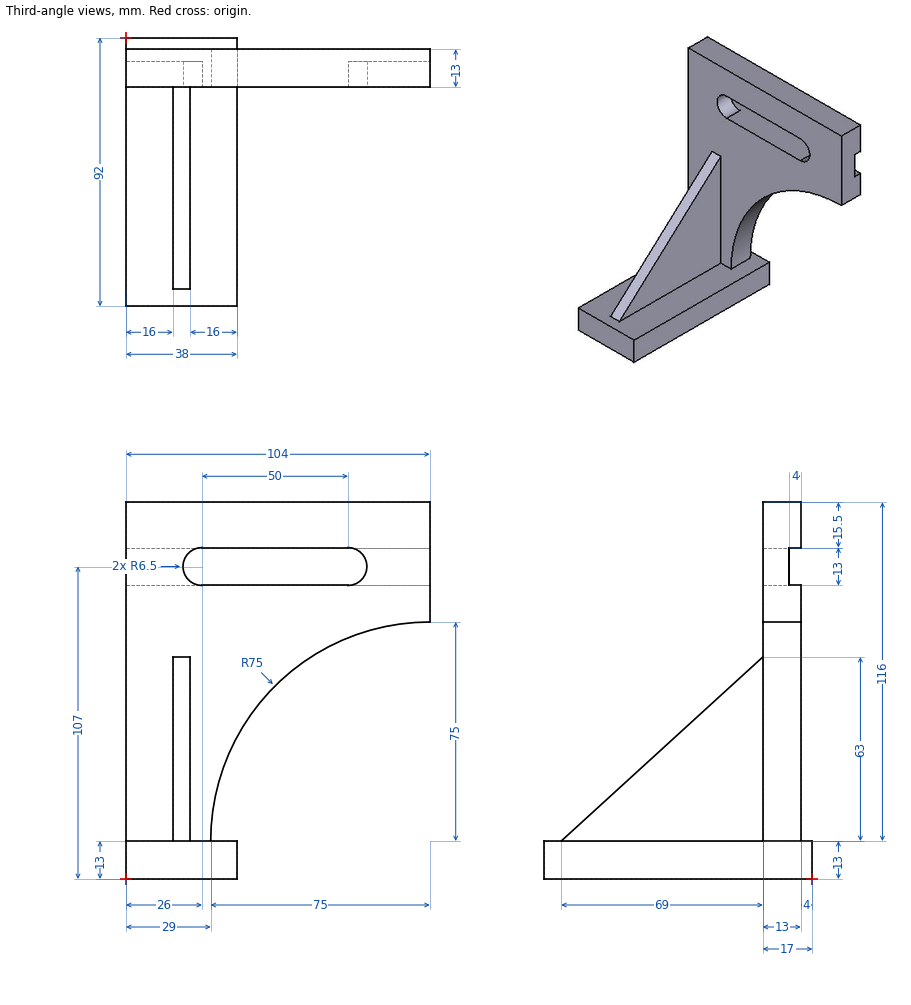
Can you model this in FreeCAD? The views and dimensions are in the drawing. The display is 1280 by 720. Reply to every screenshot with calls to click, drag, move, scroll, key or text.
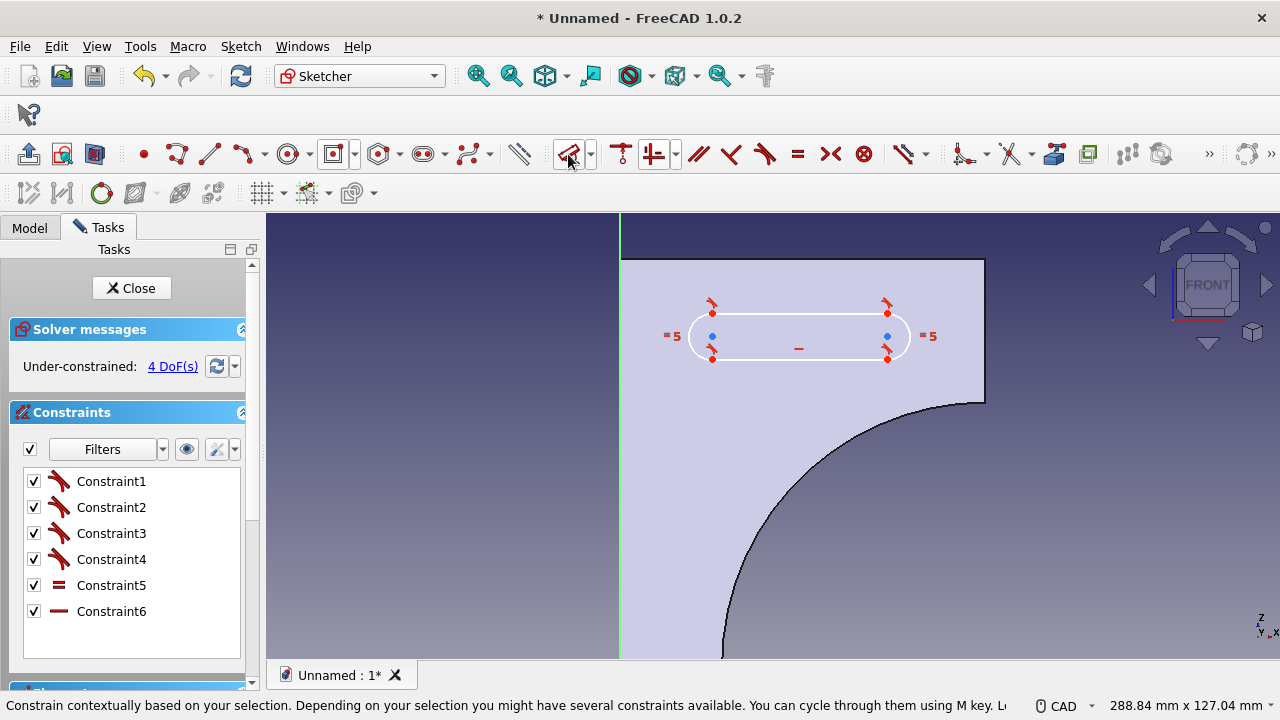
scroll(693, 323, up, 3)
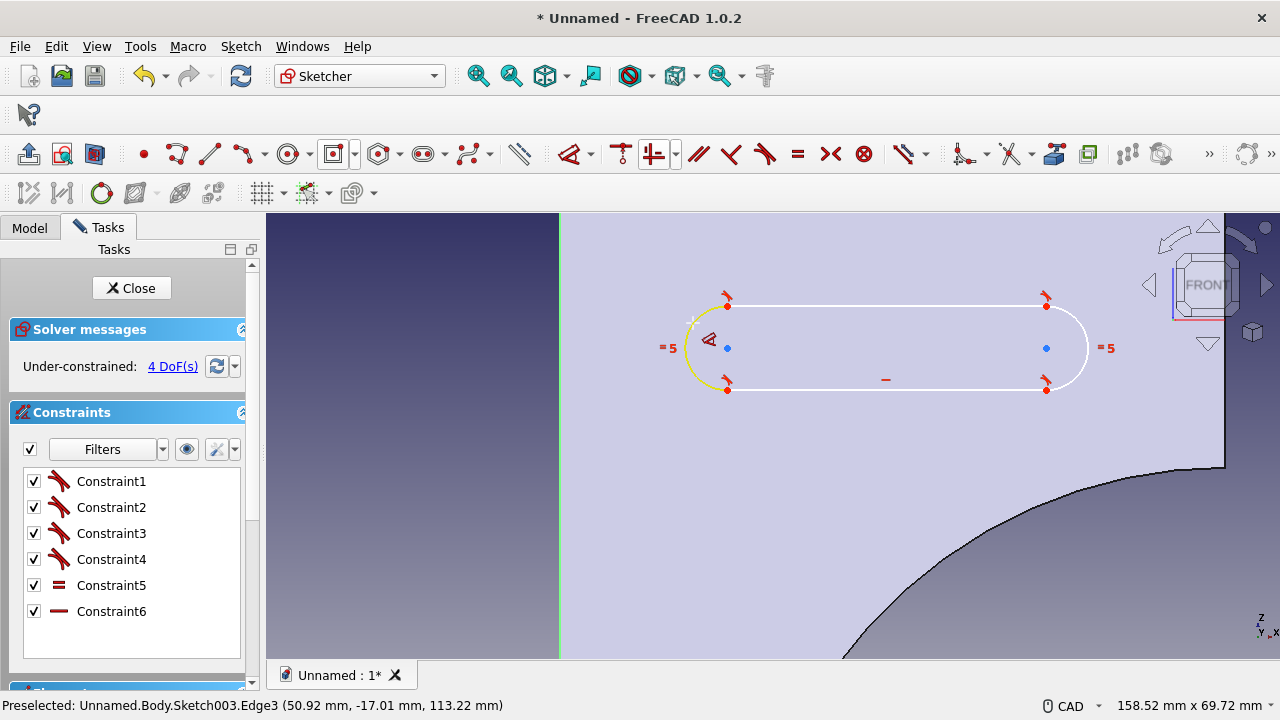
click(693, 324)
click(667, 305)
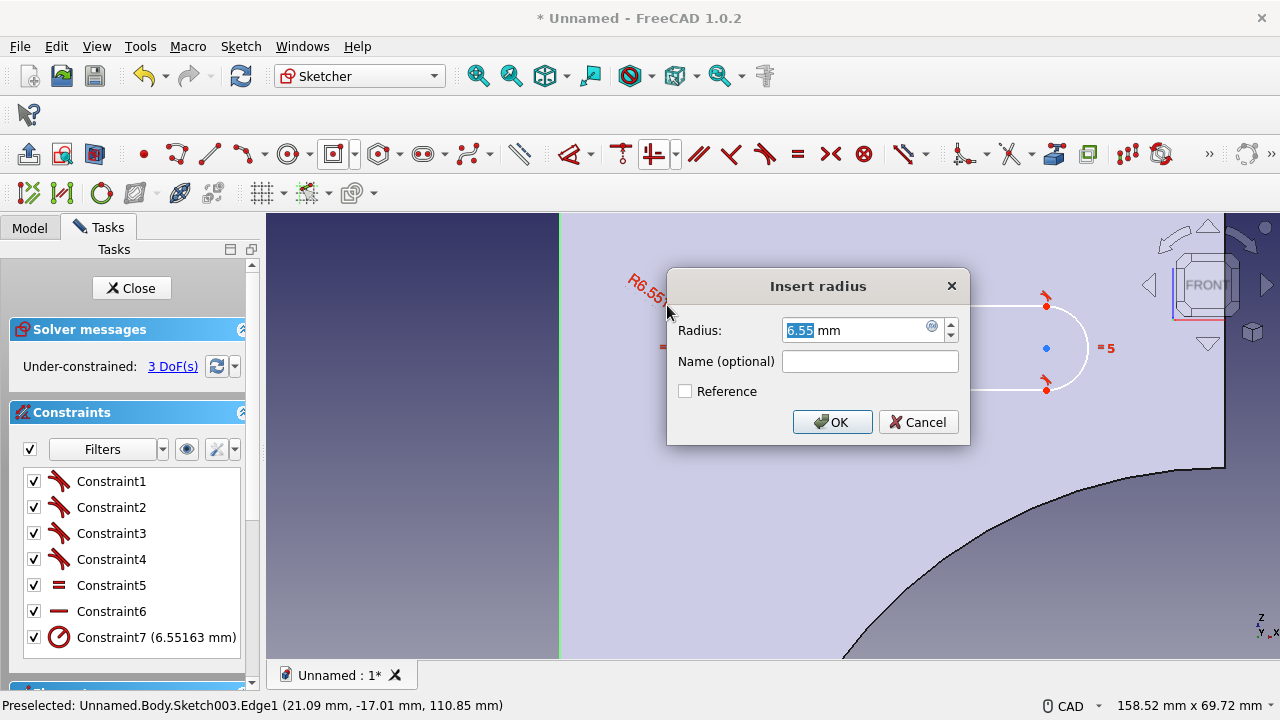
text(6.5)
key(Return)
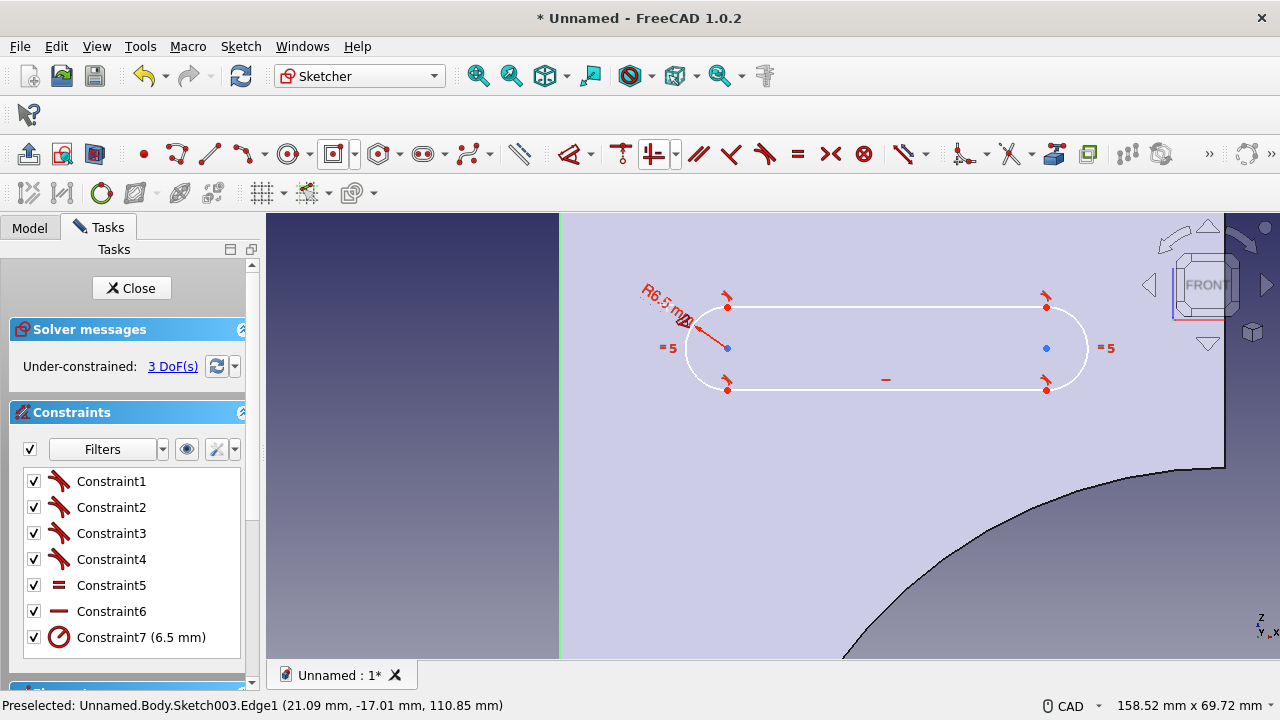
click(823, 307)
click(887, 273)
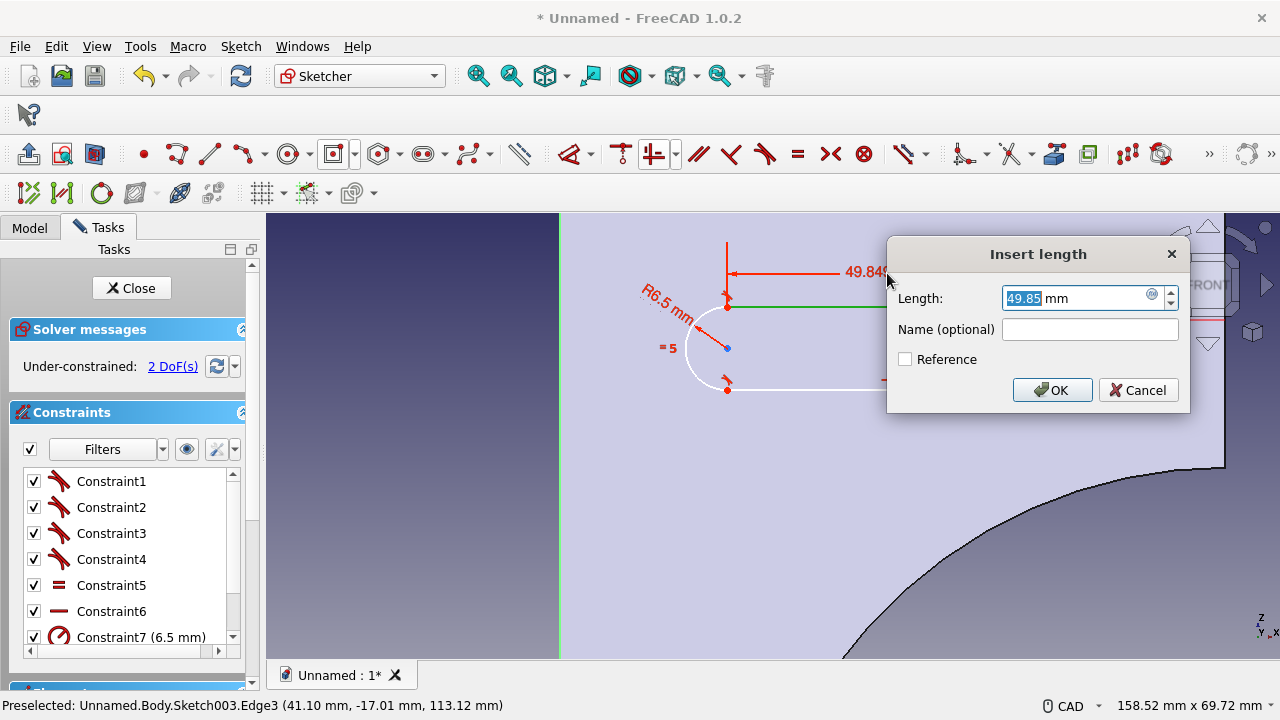
text(50)
key(Return)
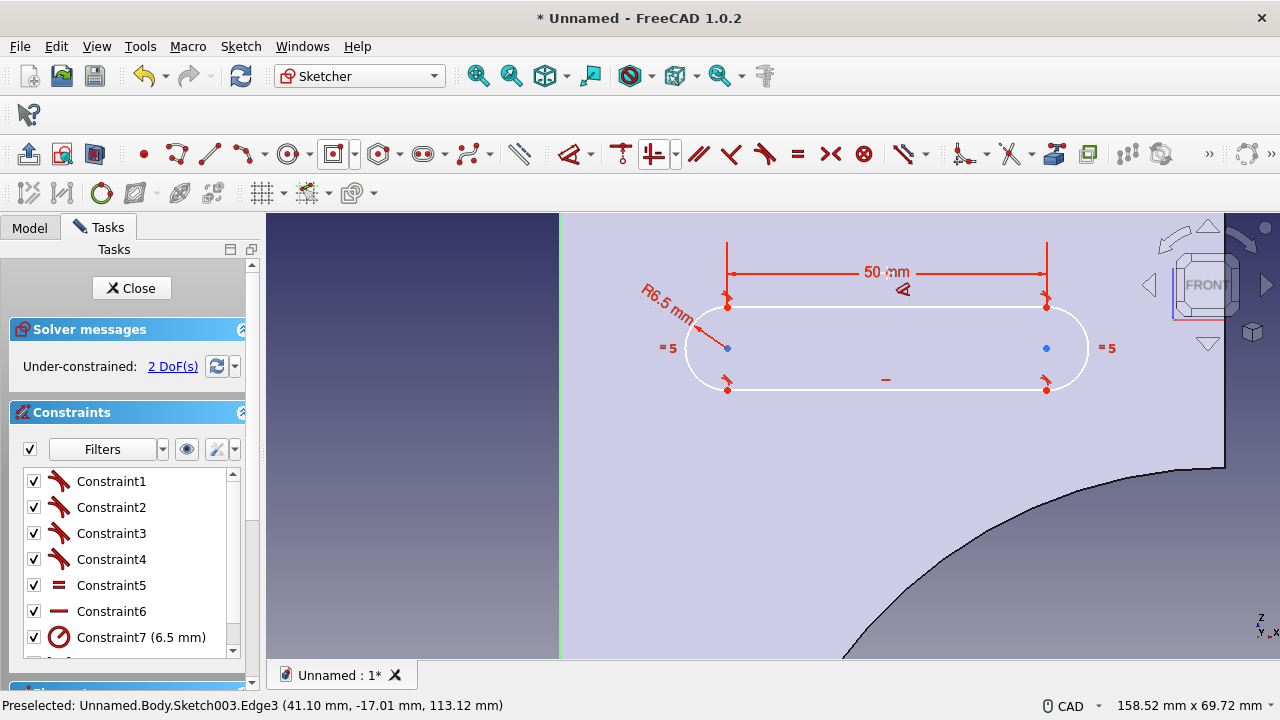
click(727, 307)
click(644, 273)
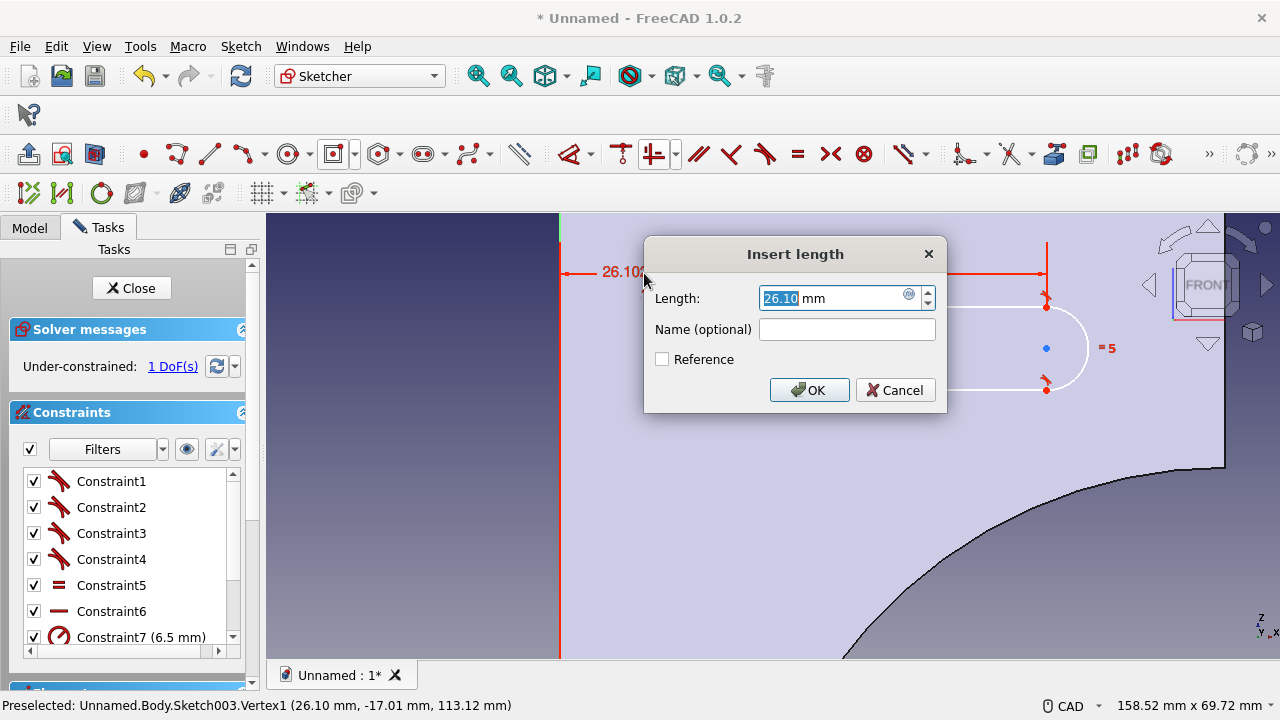
text(26)
key(Return)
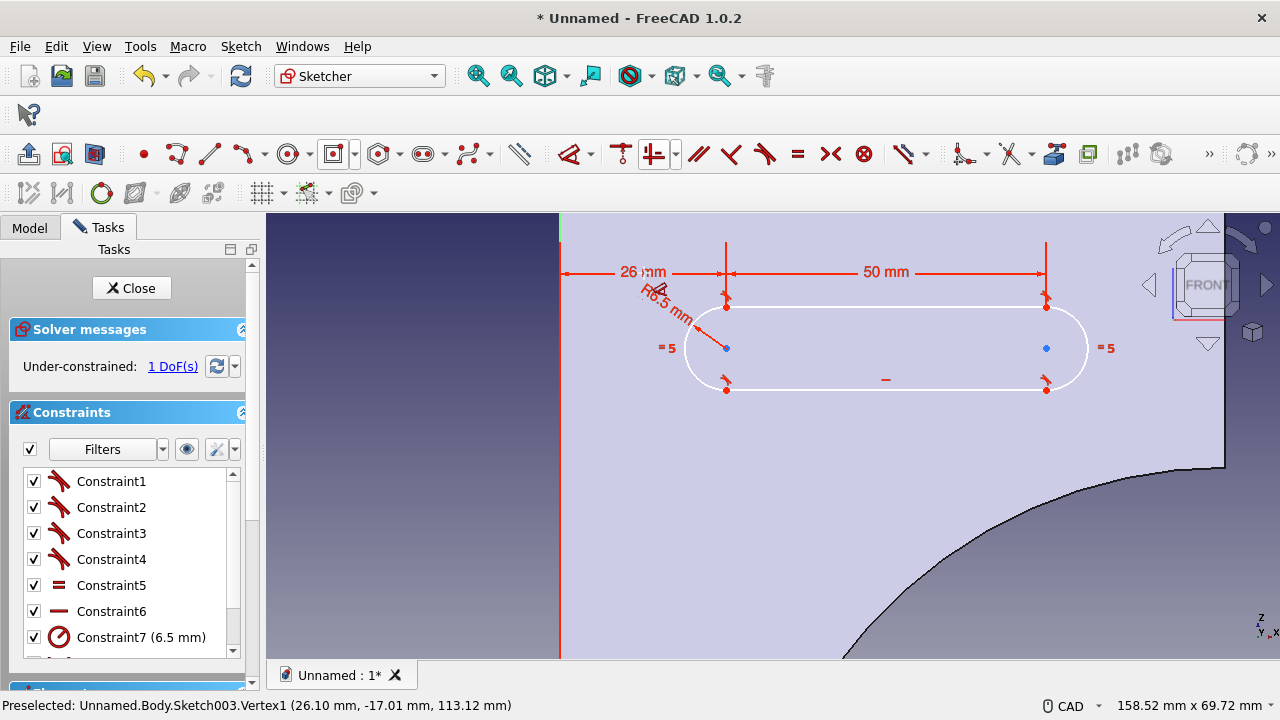
click(726, 349)
click(526, 490)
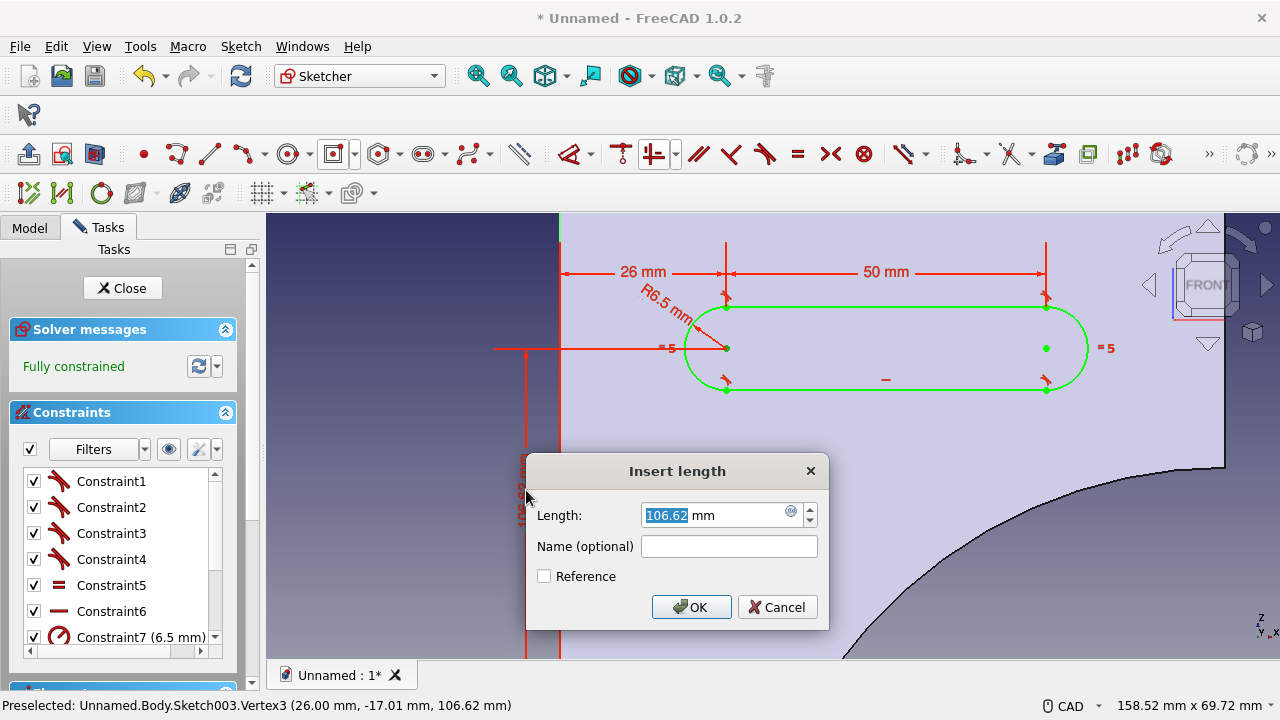
text(107)
key(Return)
key(Escape)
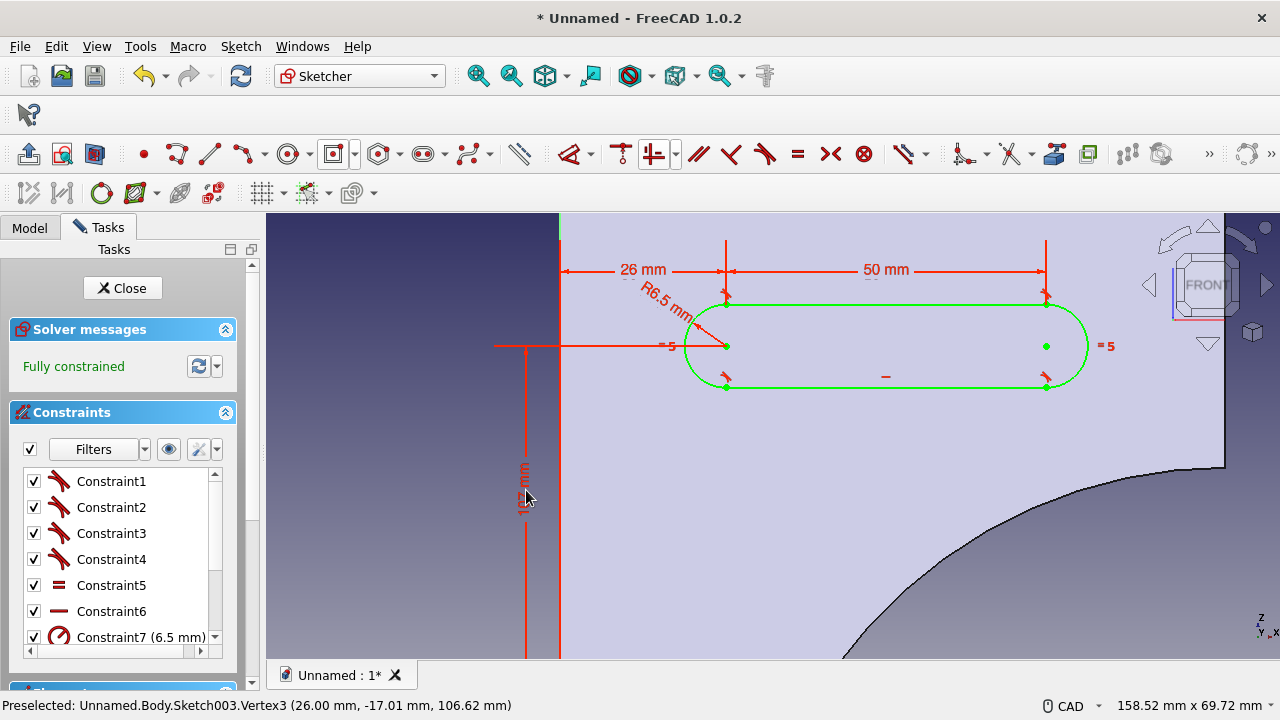
click(123, 288)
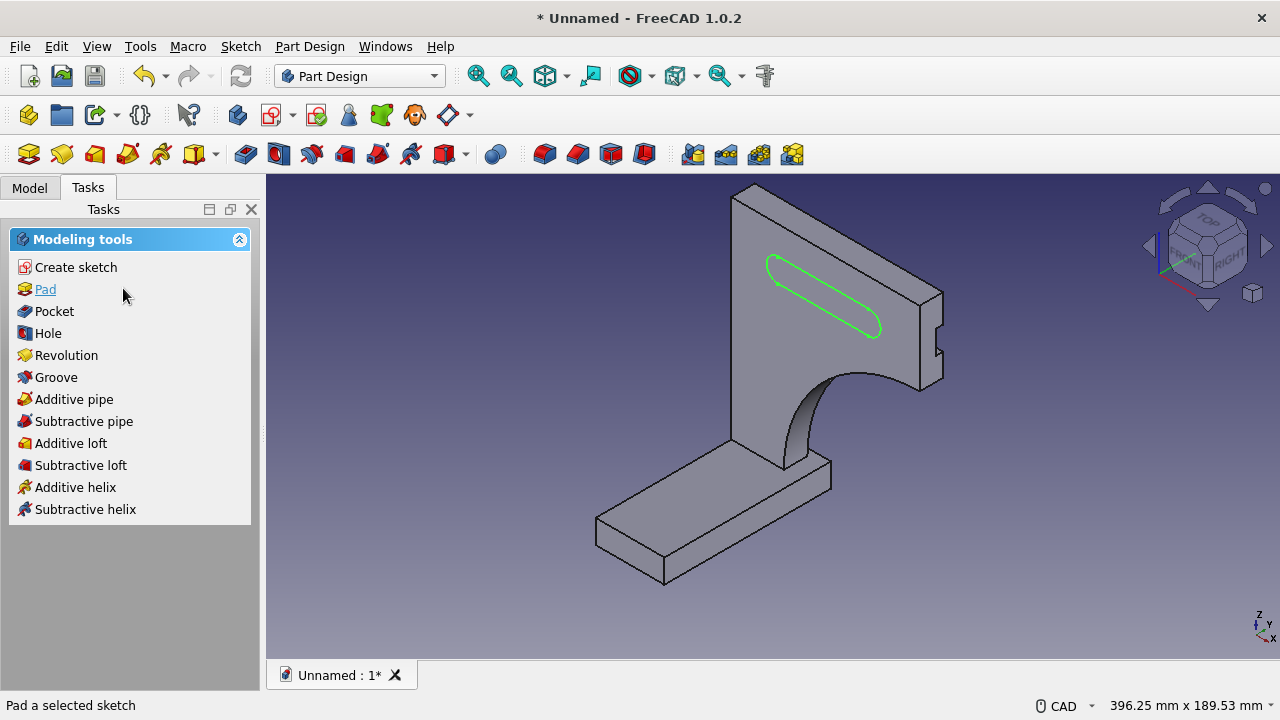
click(246, 154)